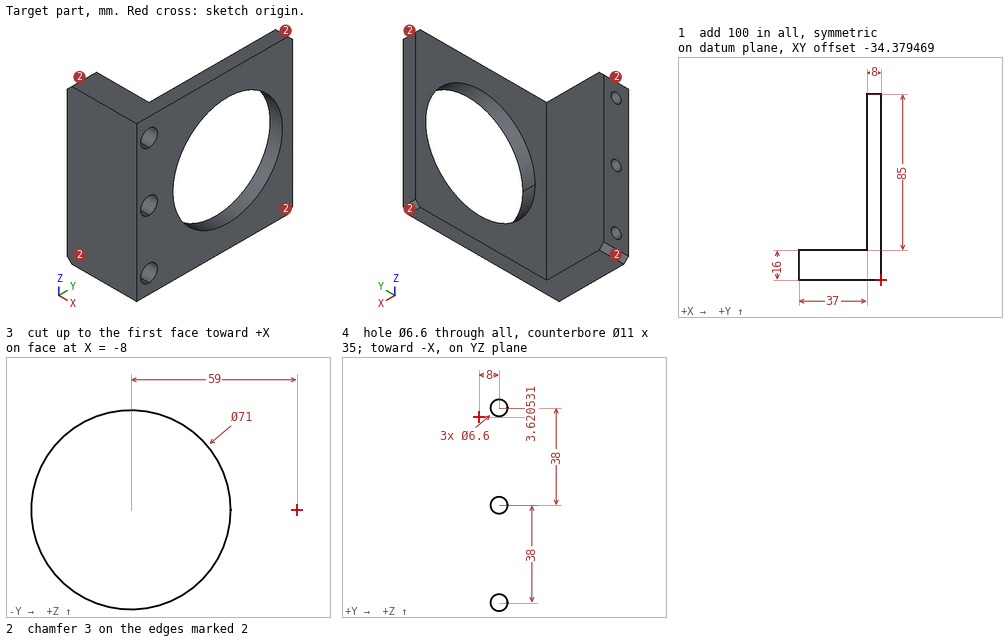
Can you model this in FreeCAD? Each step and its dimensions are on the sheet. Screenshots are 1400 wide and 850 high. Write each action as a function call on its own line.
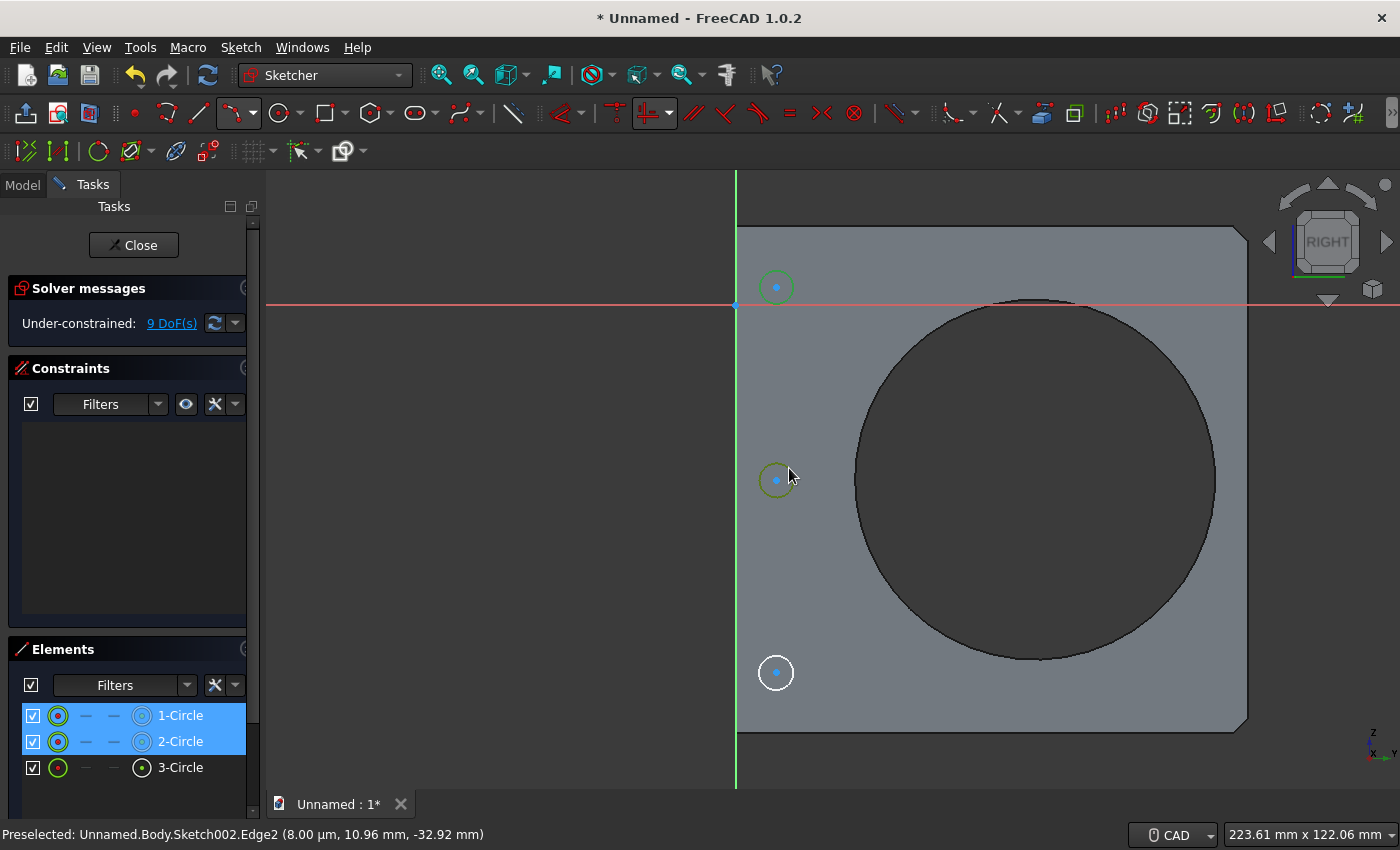
click(788, 661)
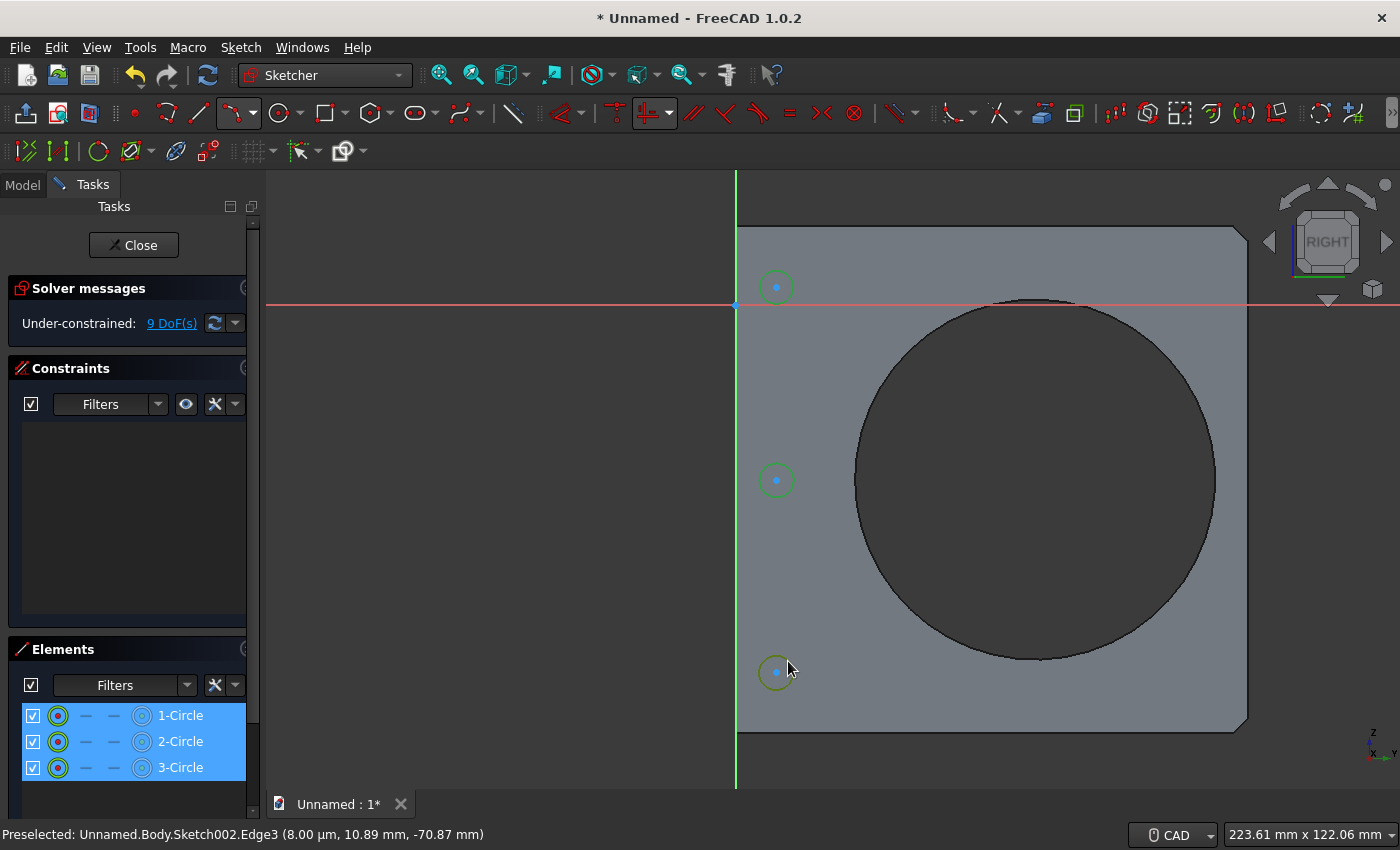
click(790, 114)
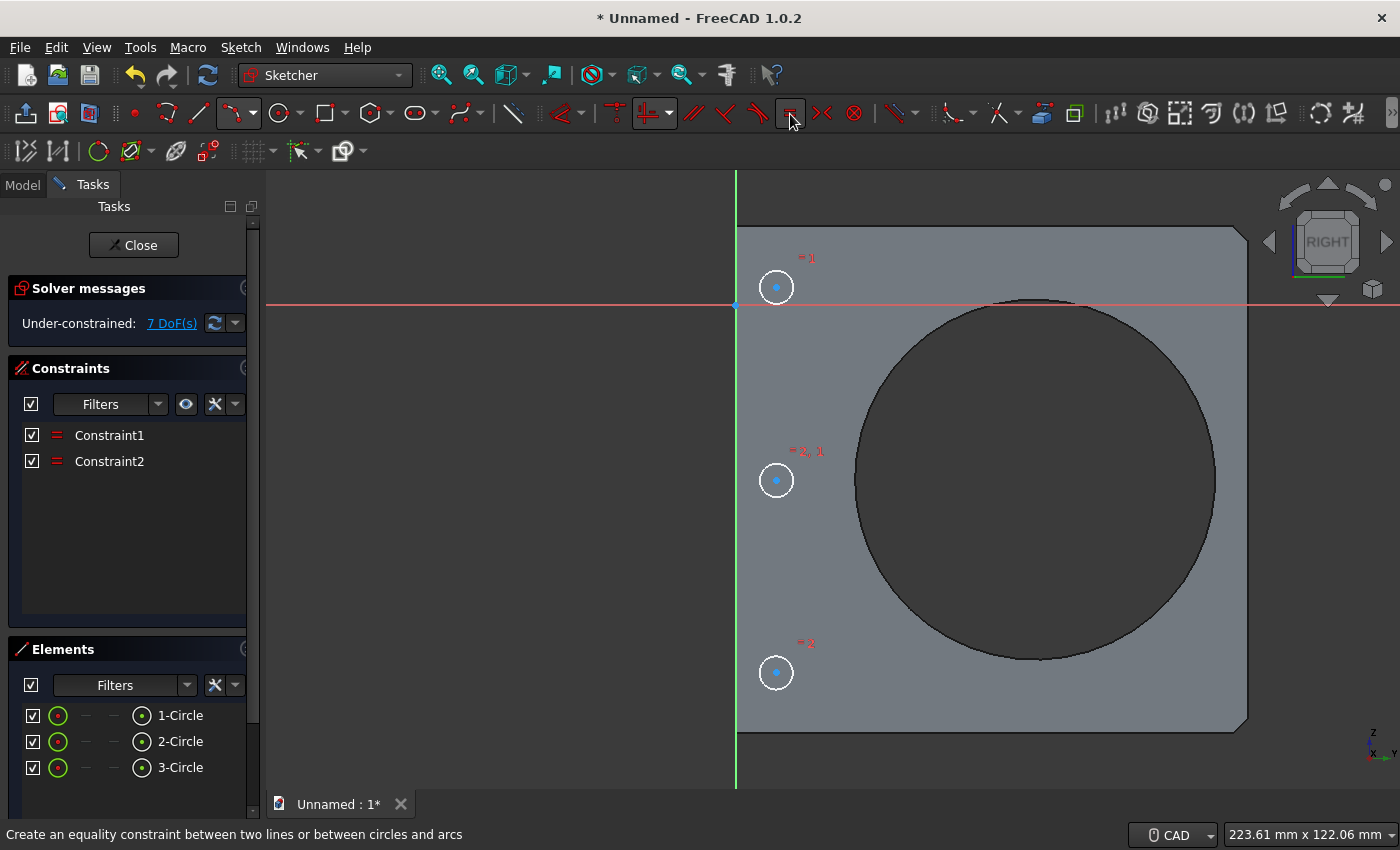
click(777, 287)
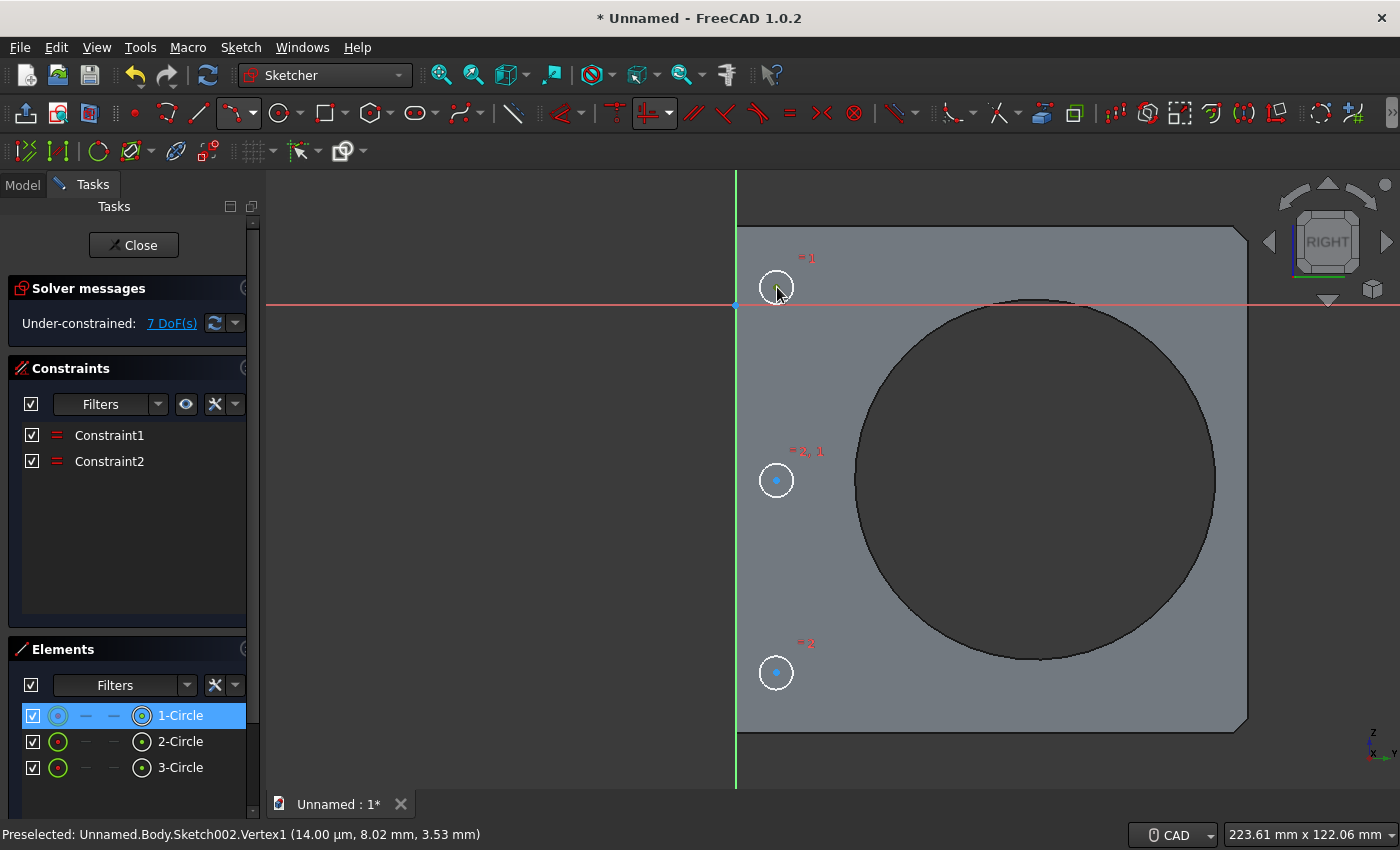
click(777, 480)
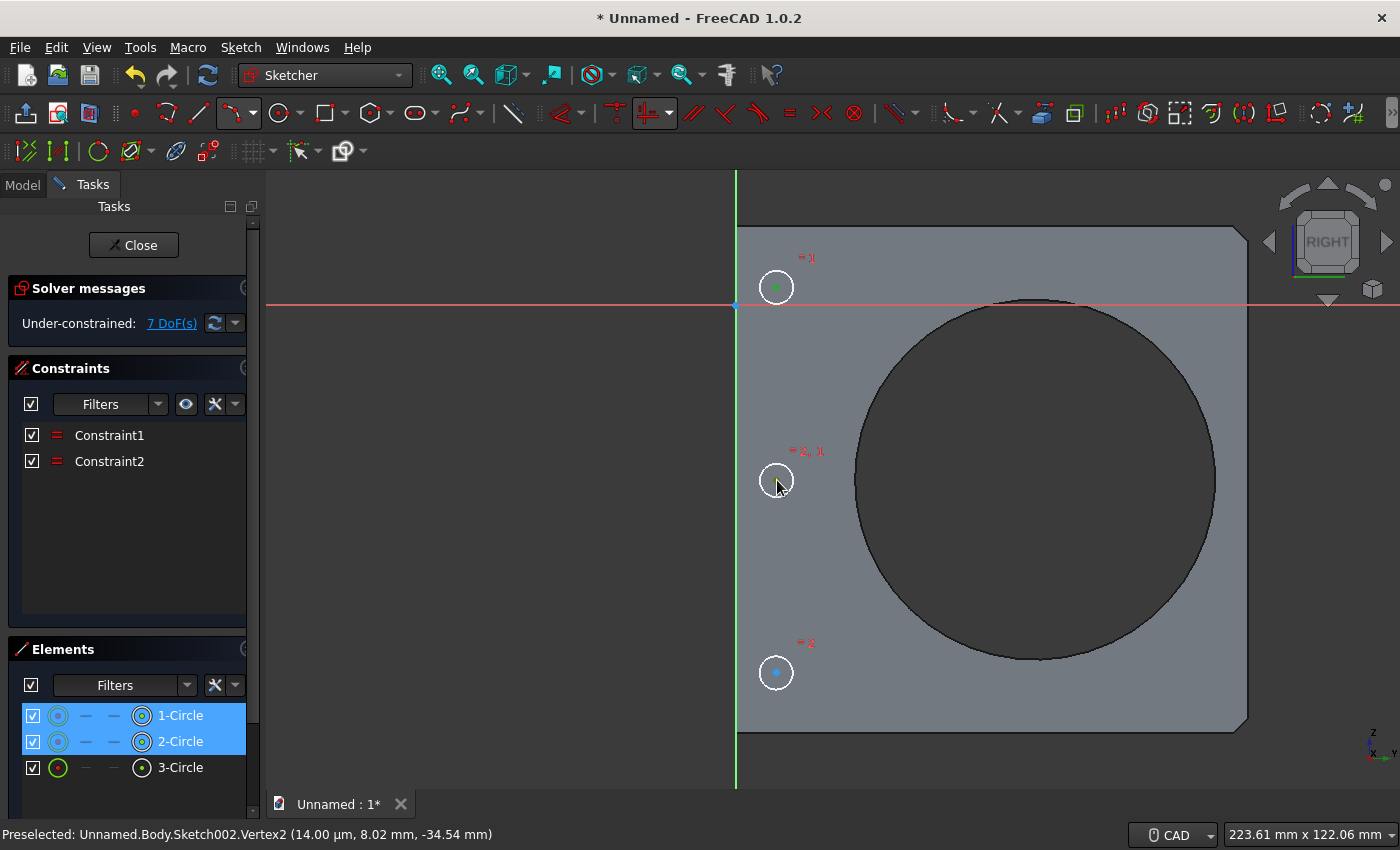
click(672, 114)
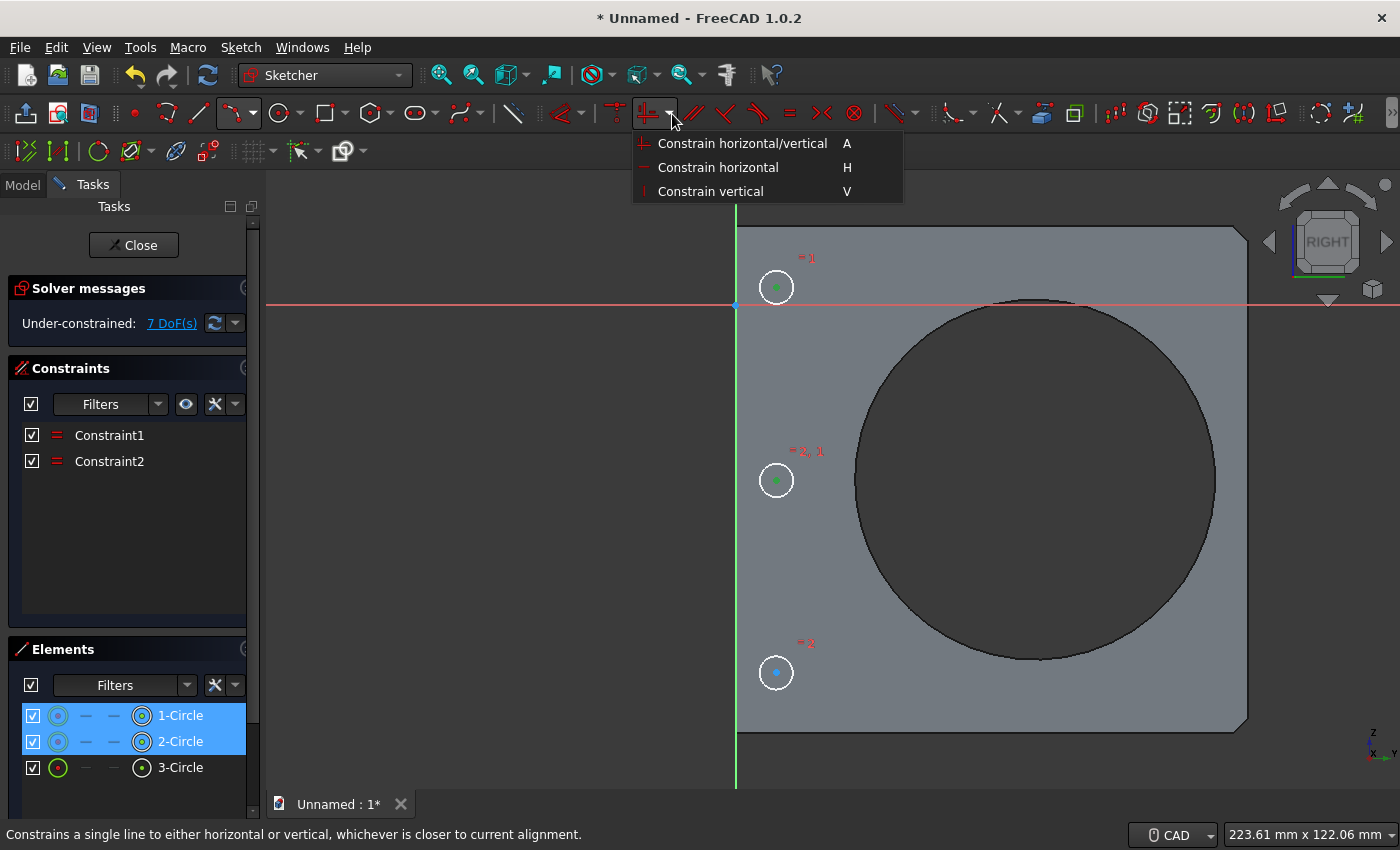
click(768, 191)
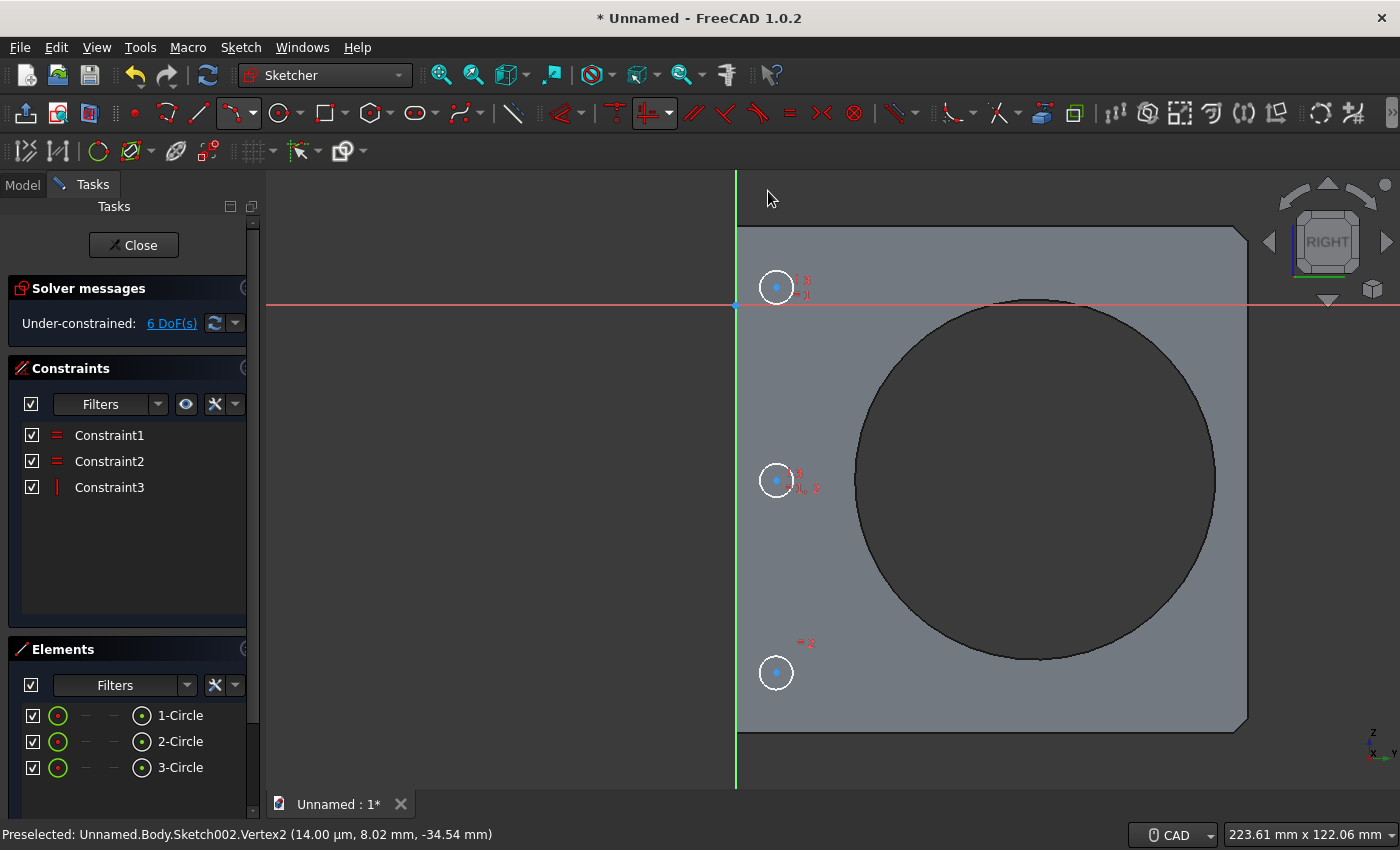
click(777, 480)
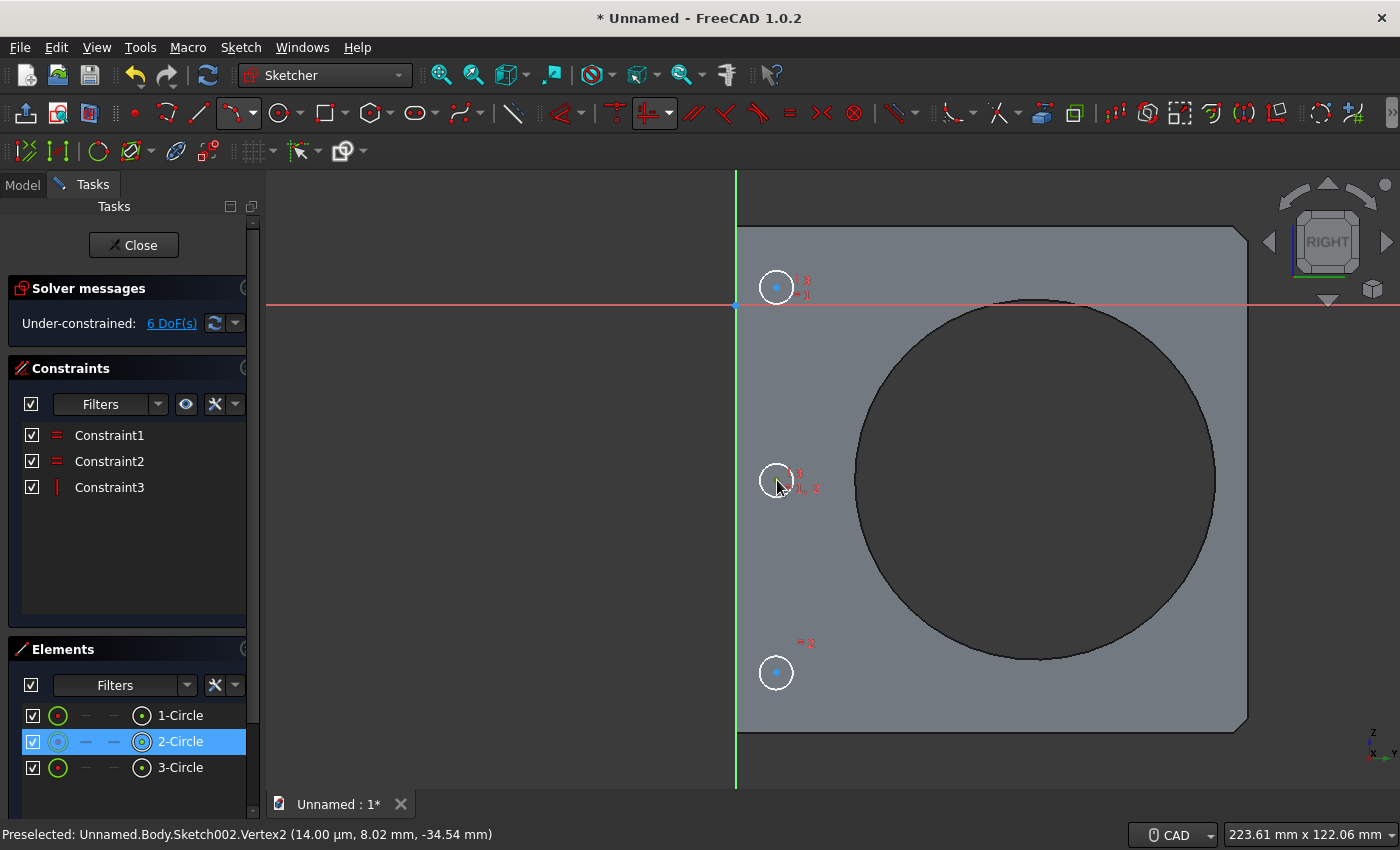
click(776, 673)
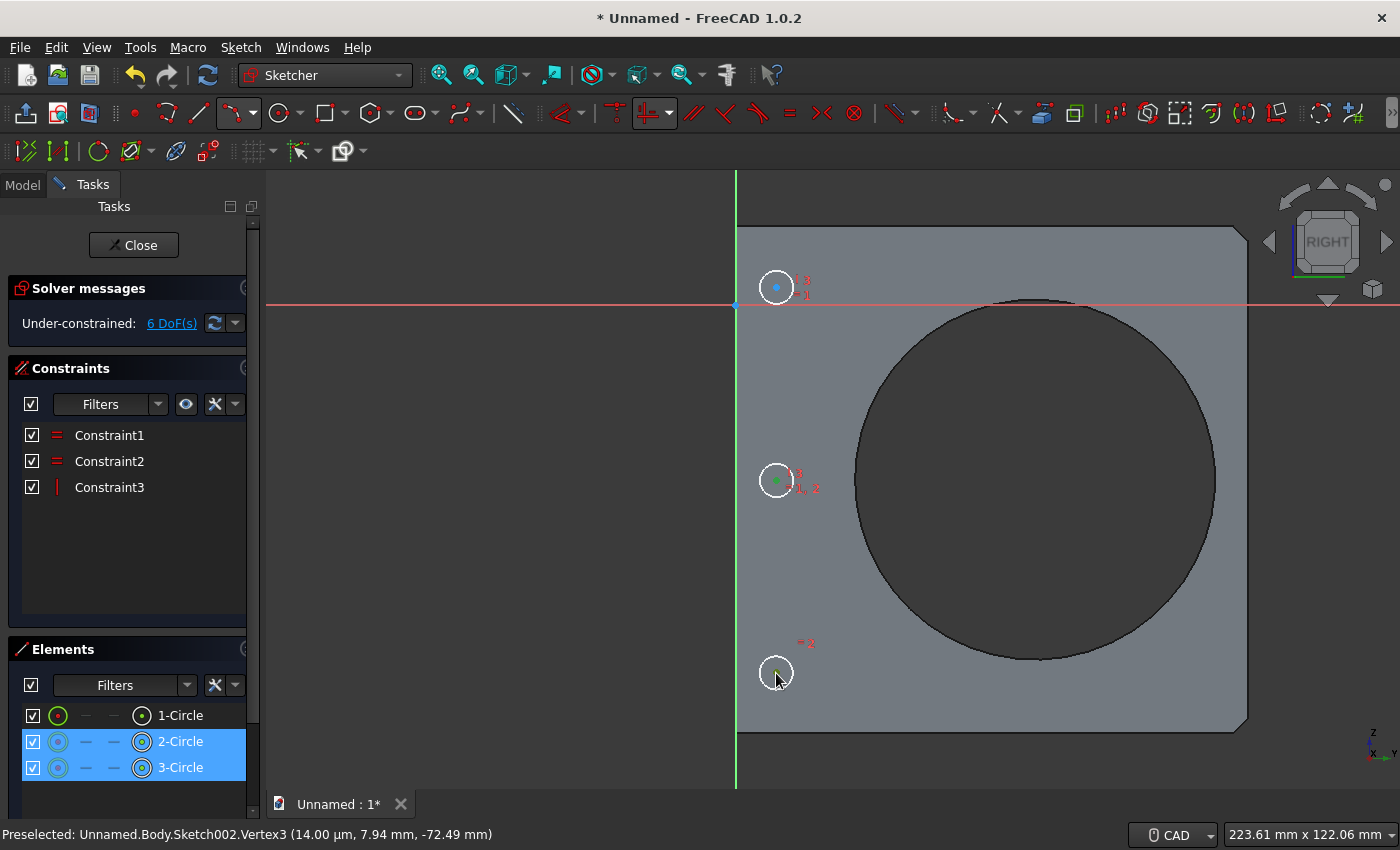
click(672, 114)